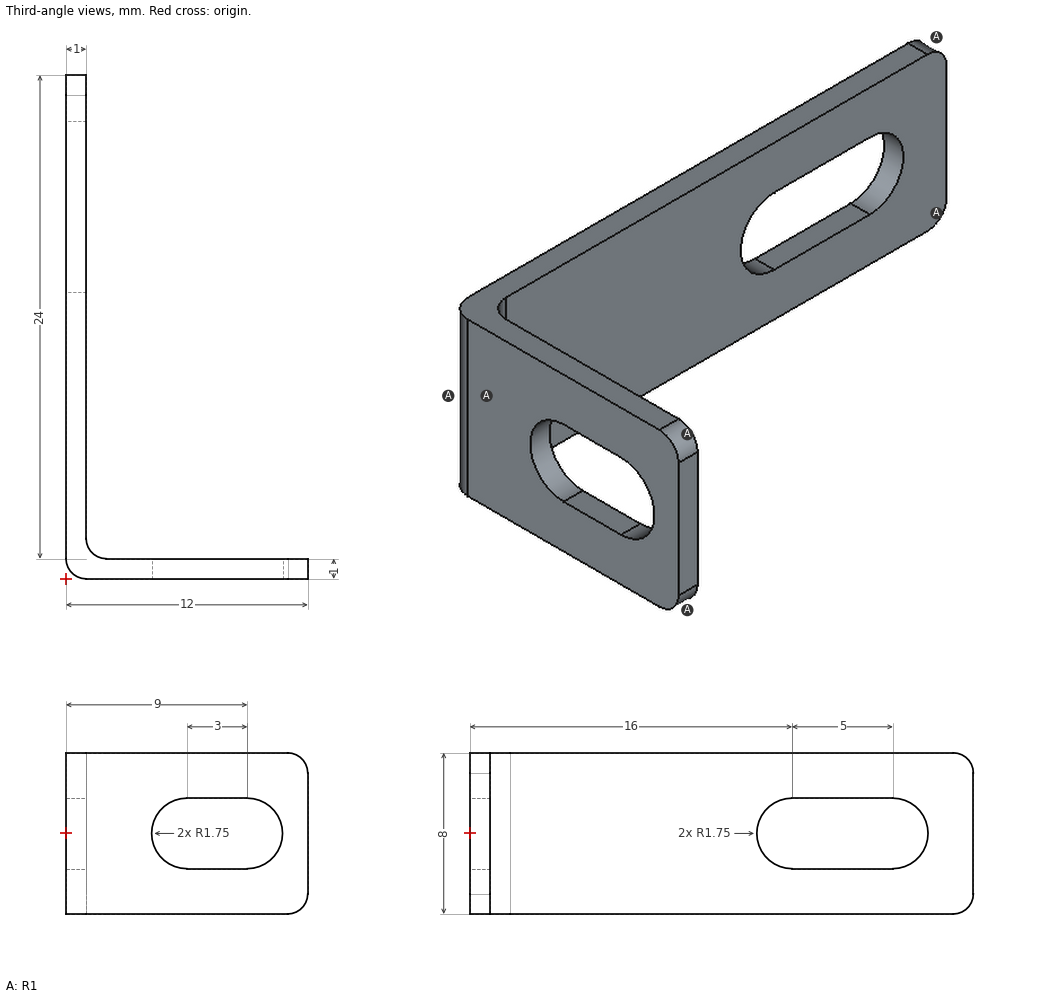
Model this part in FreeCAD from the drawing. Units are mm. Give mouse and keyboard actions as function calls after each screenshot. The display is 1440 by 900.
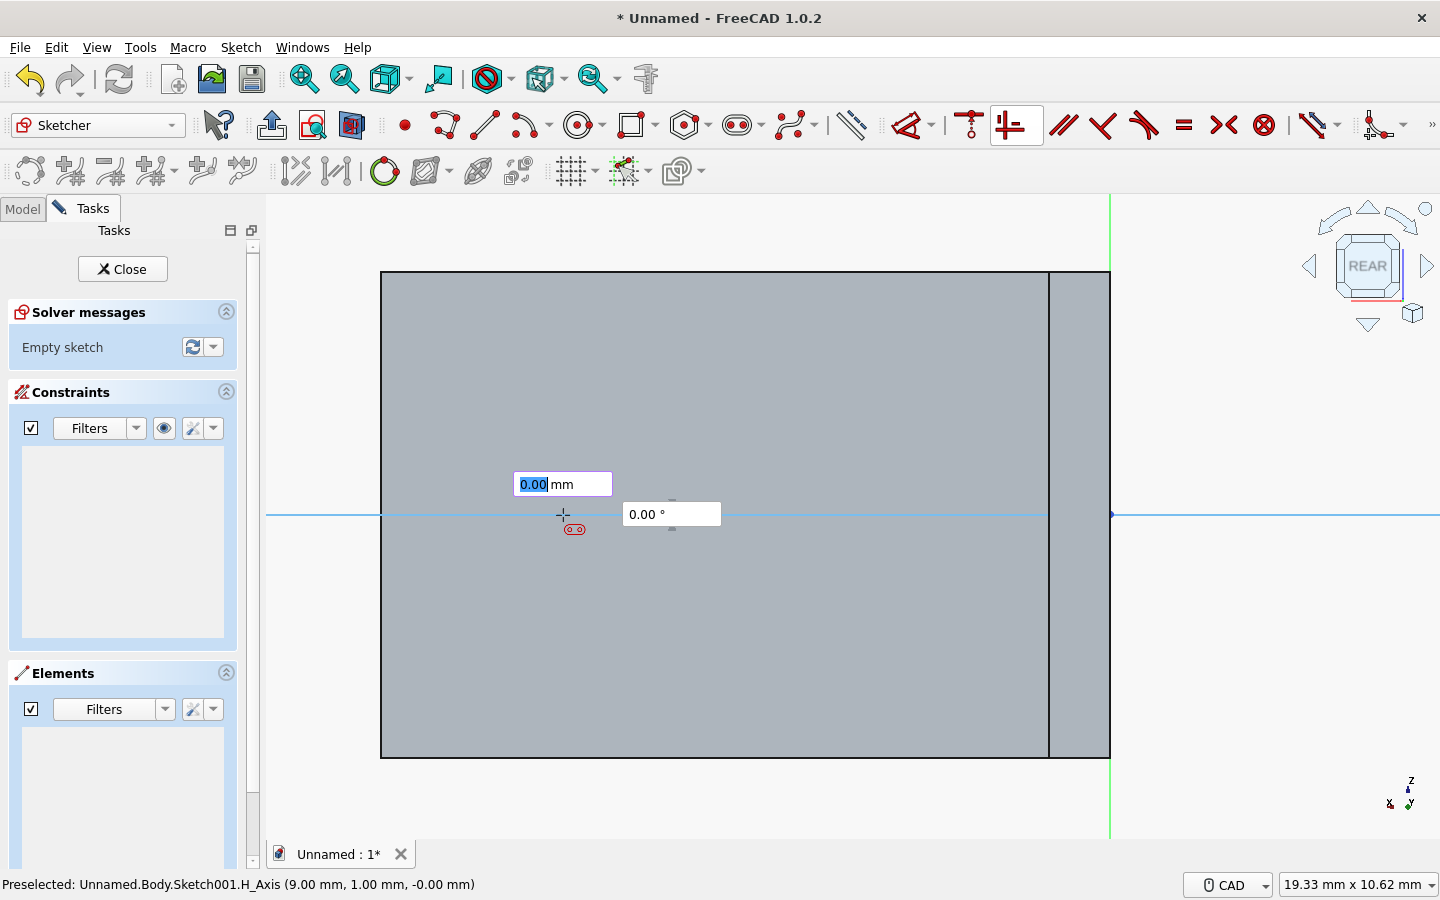
click(746, 506)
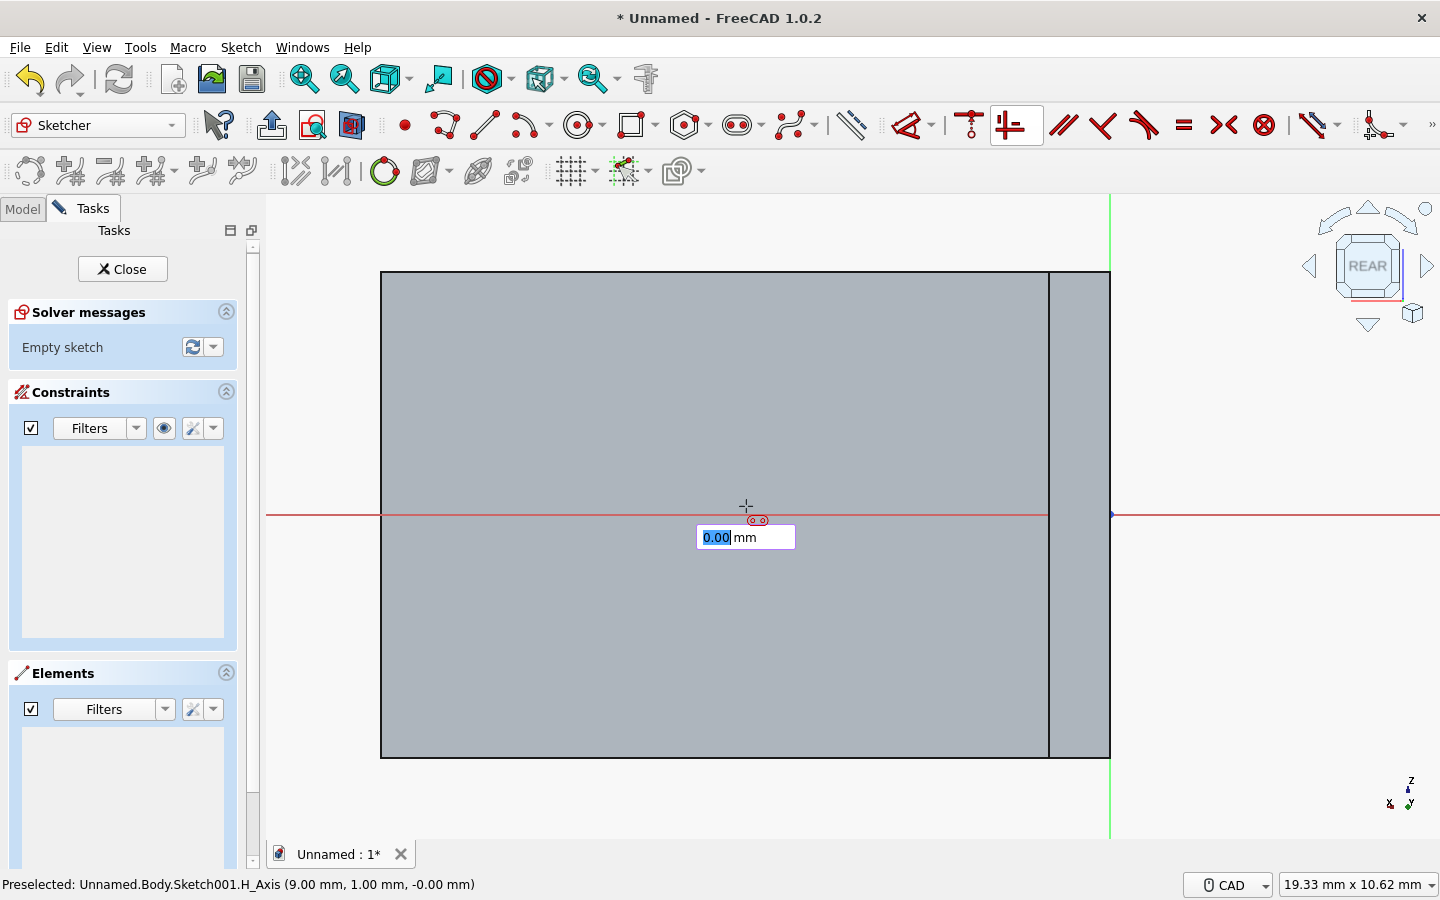
click(654, 621)
key(Escape)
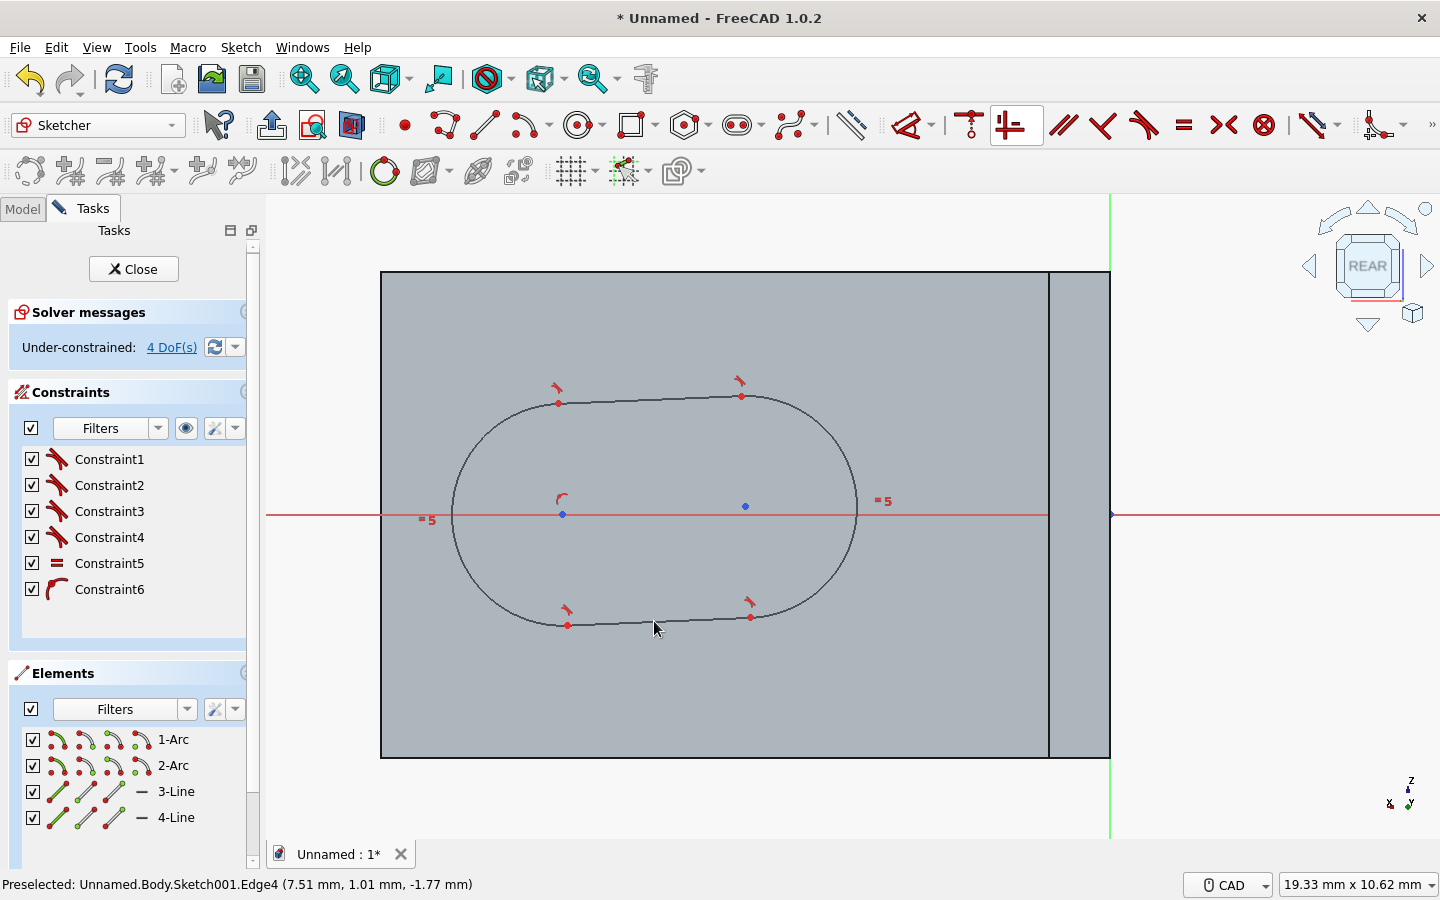
click(613, 402)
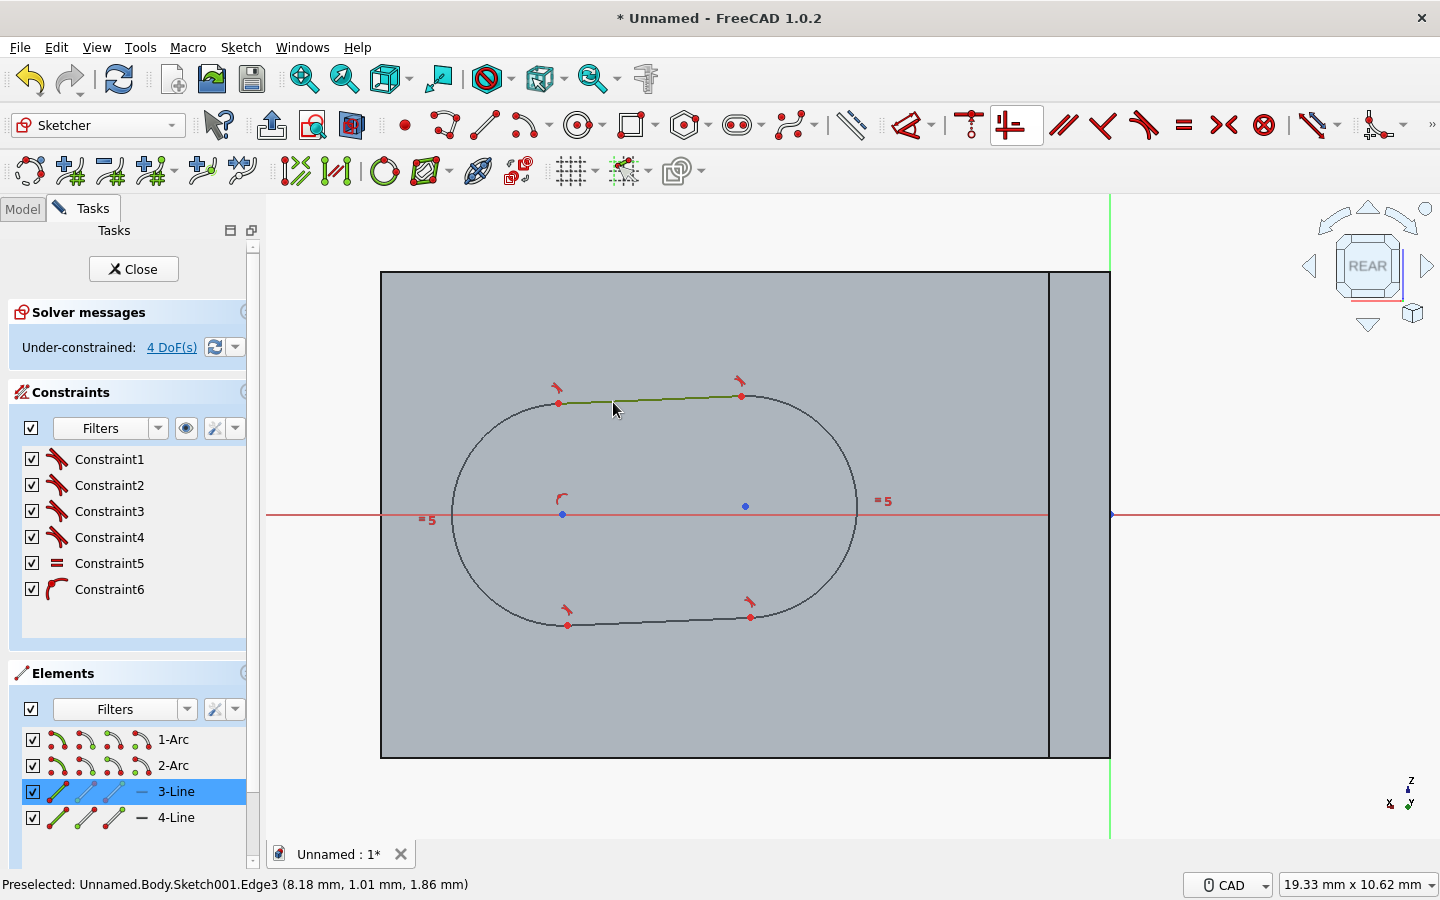
key(h)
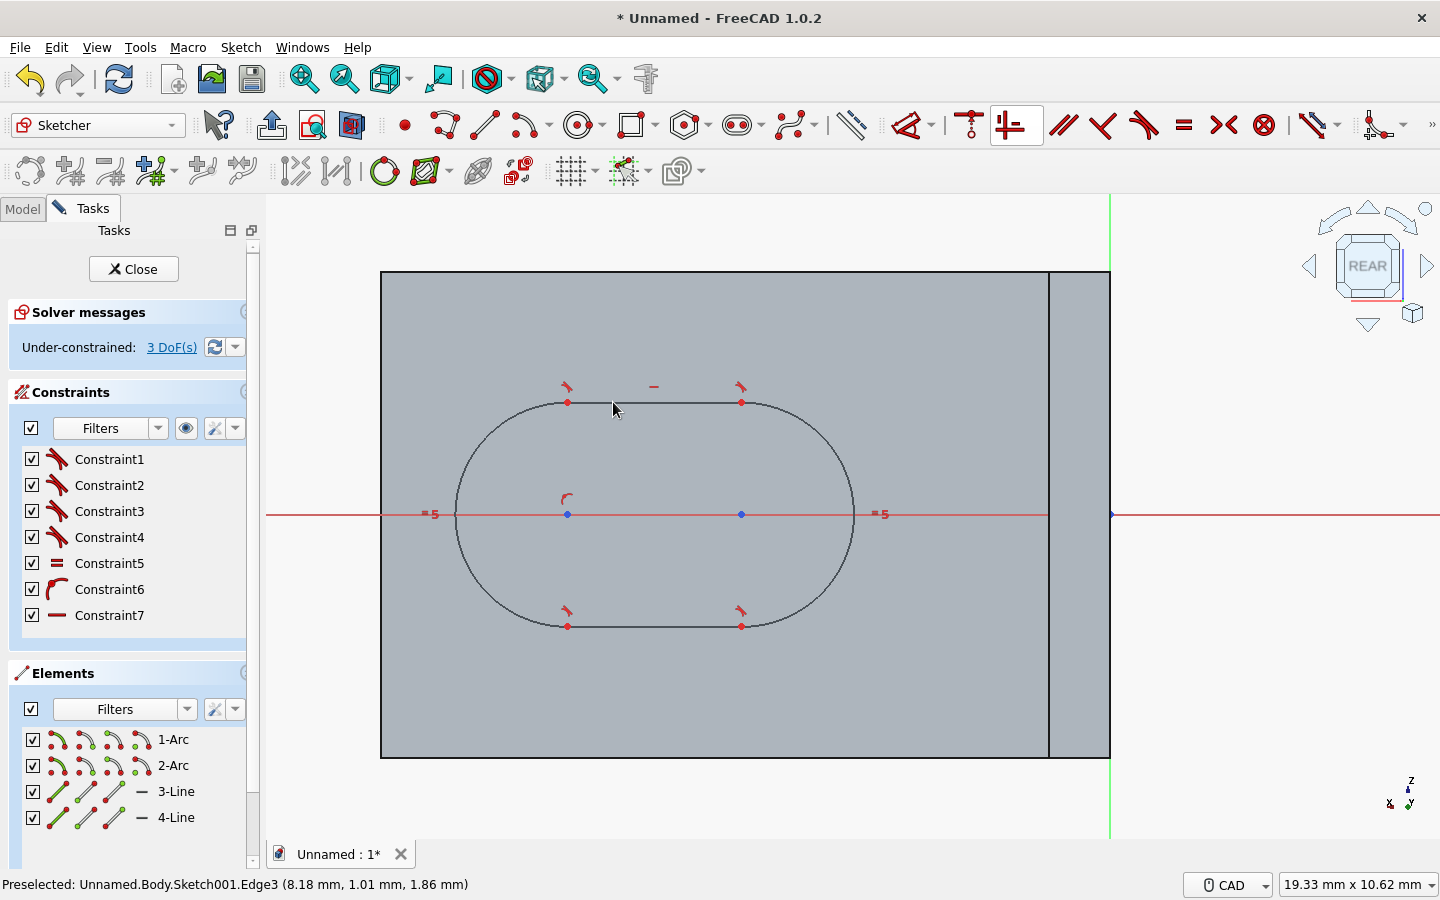
key(d)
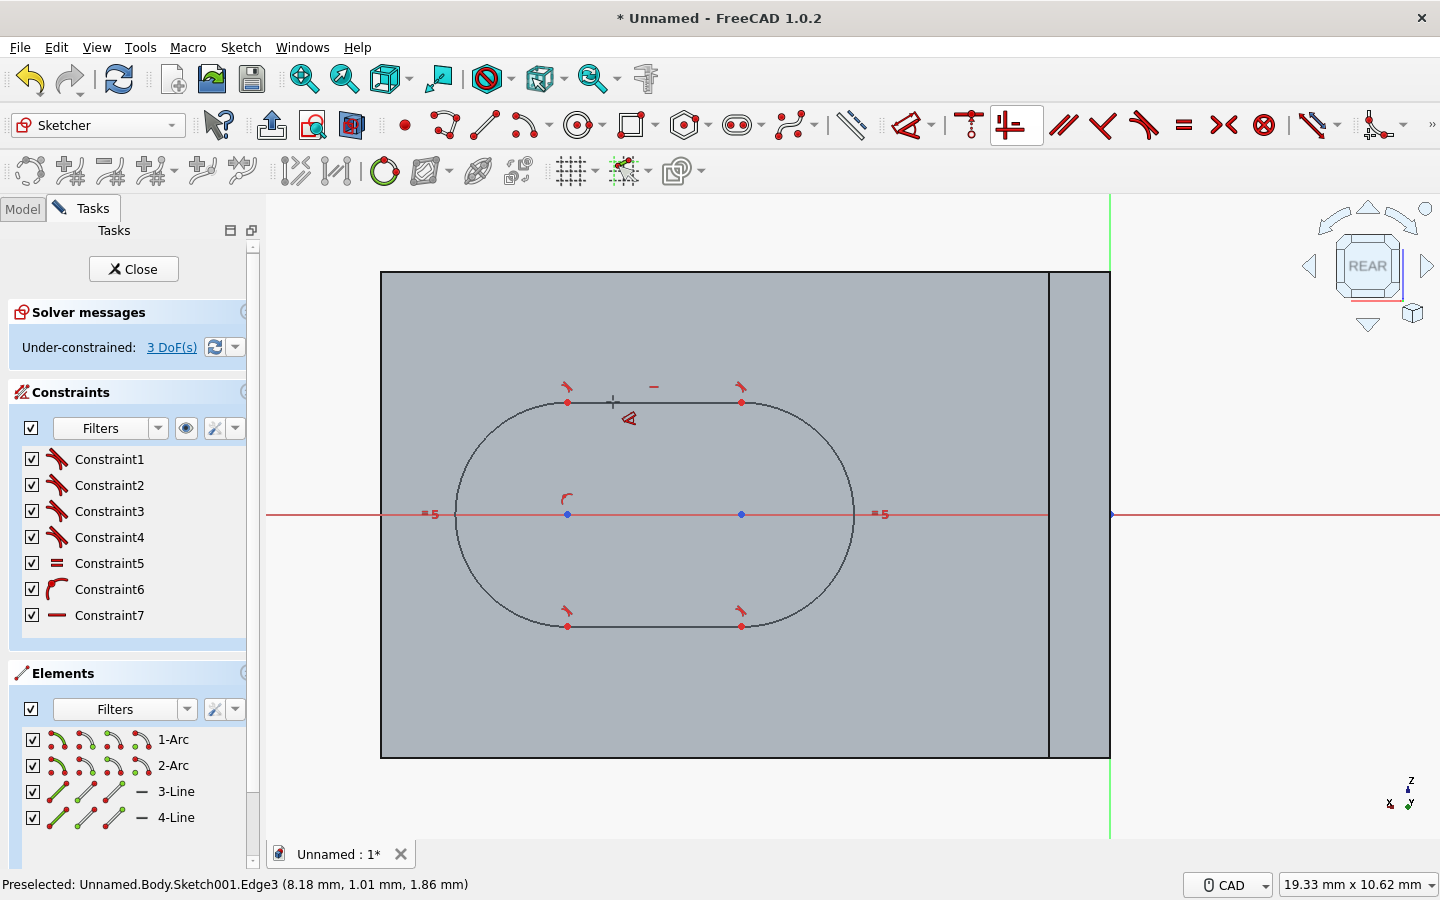
click(477, 449)
click(451, 430)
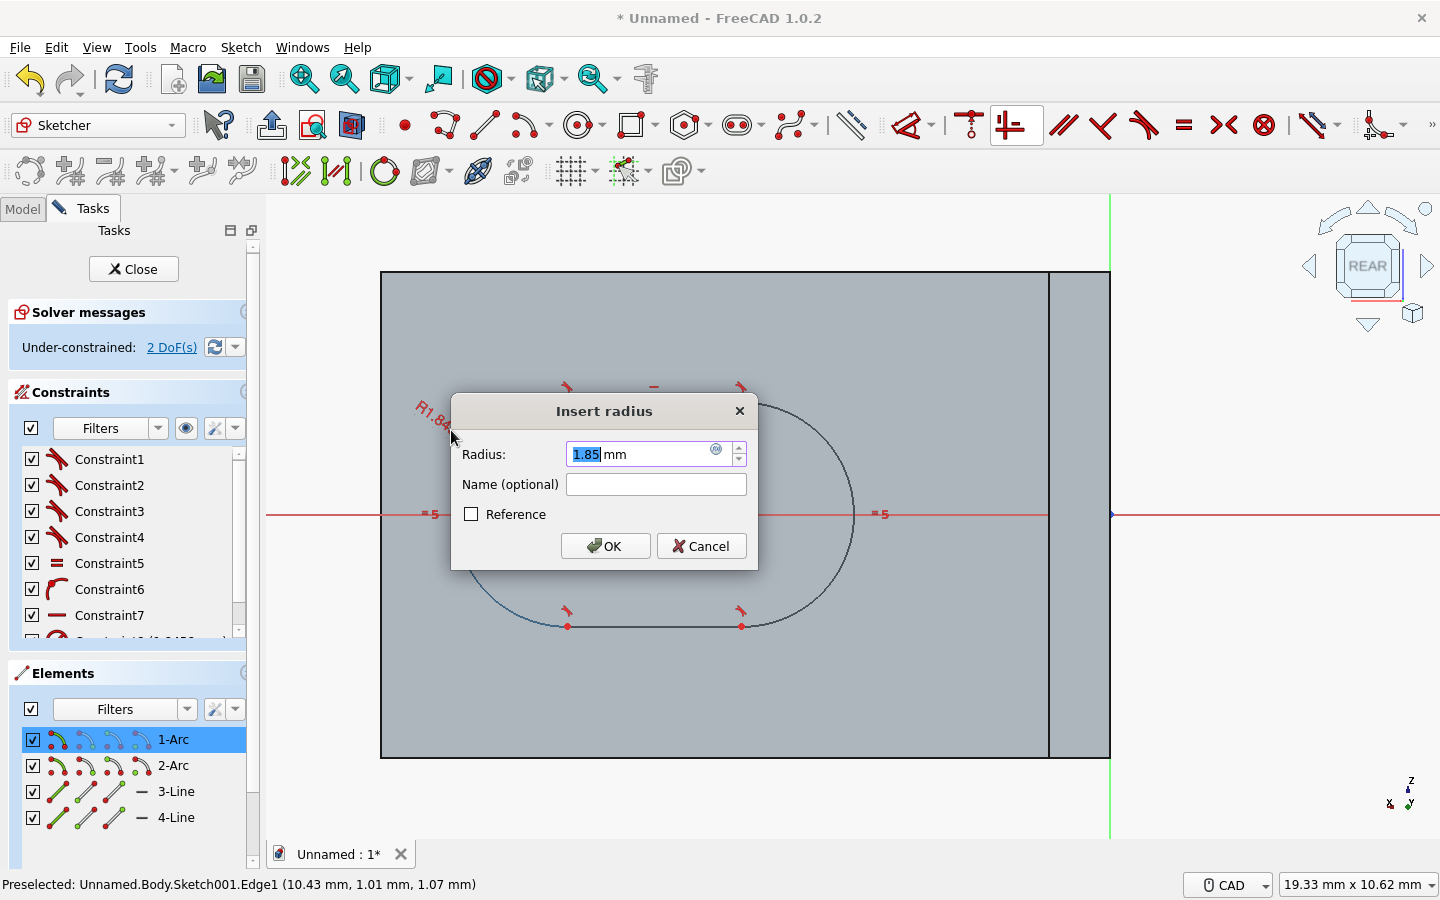
text(1.75)
key(Return)